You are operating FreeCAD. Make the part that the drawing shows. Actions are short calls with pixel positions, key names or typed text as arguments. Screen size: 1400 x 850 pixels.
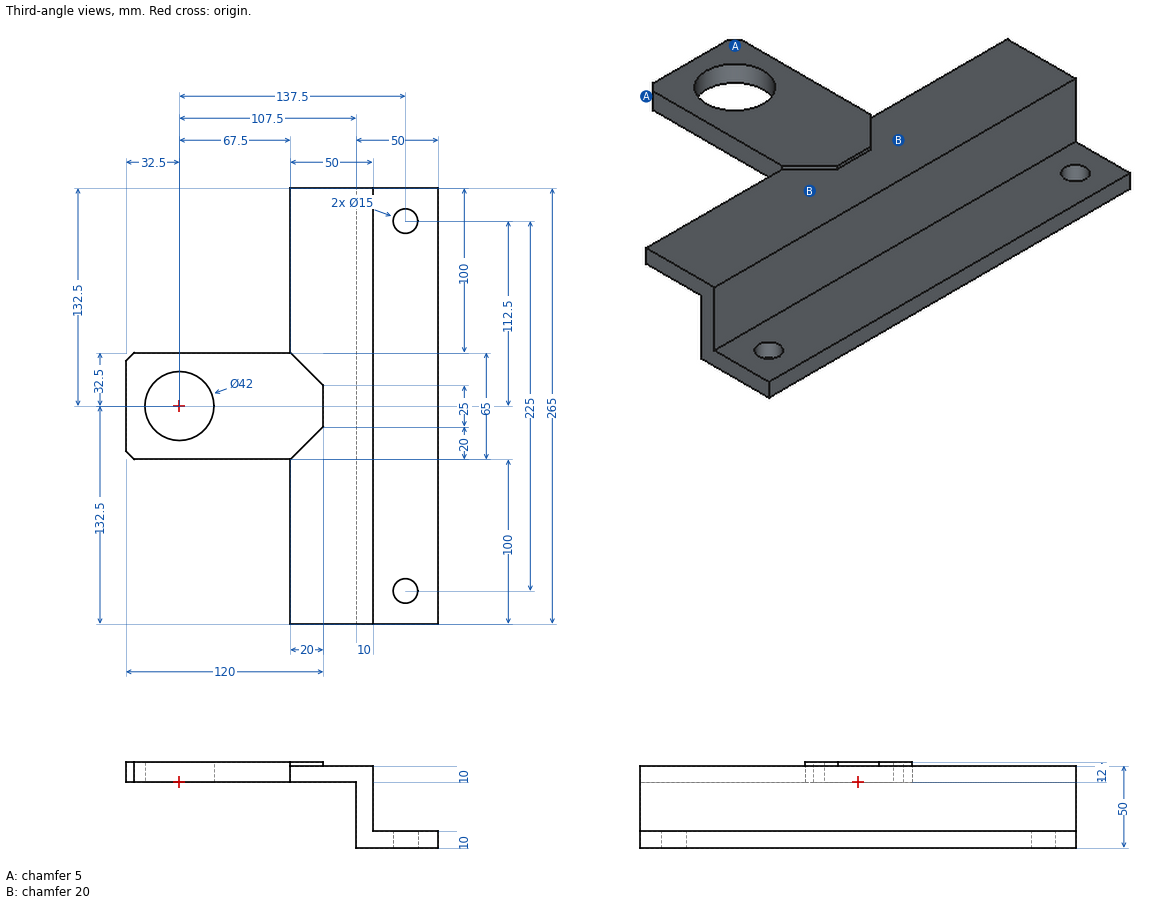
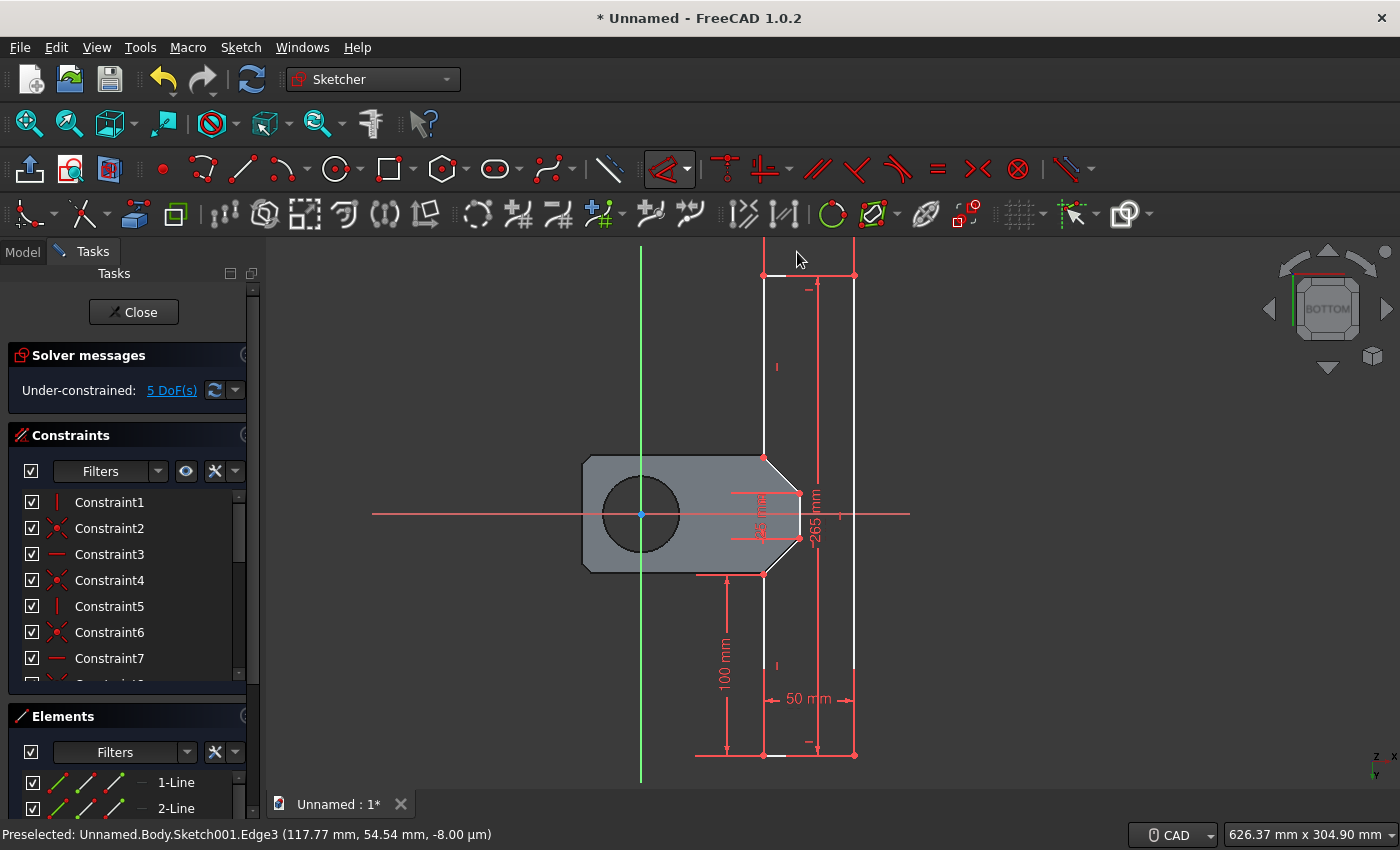
click(764, 330)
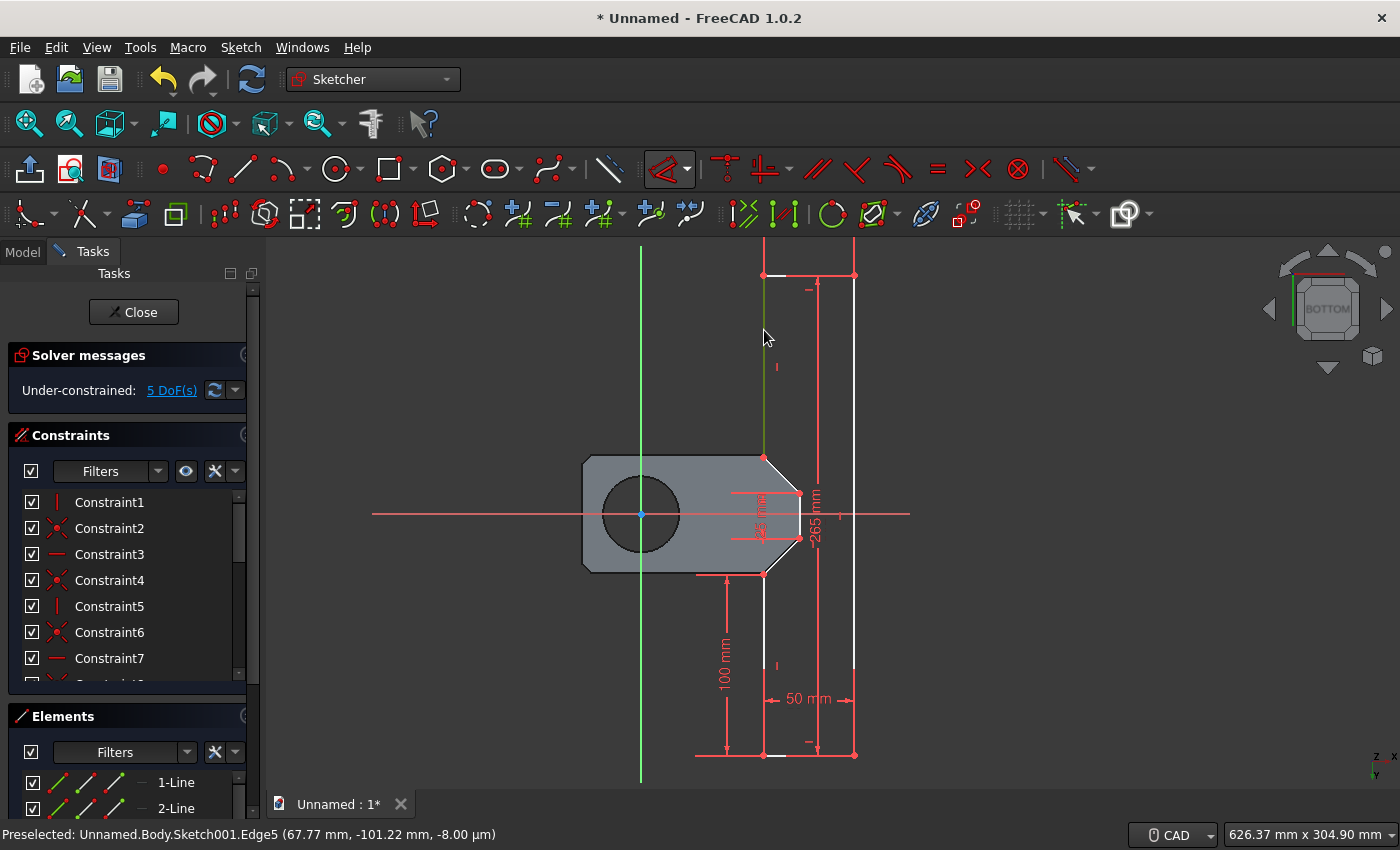
key(i)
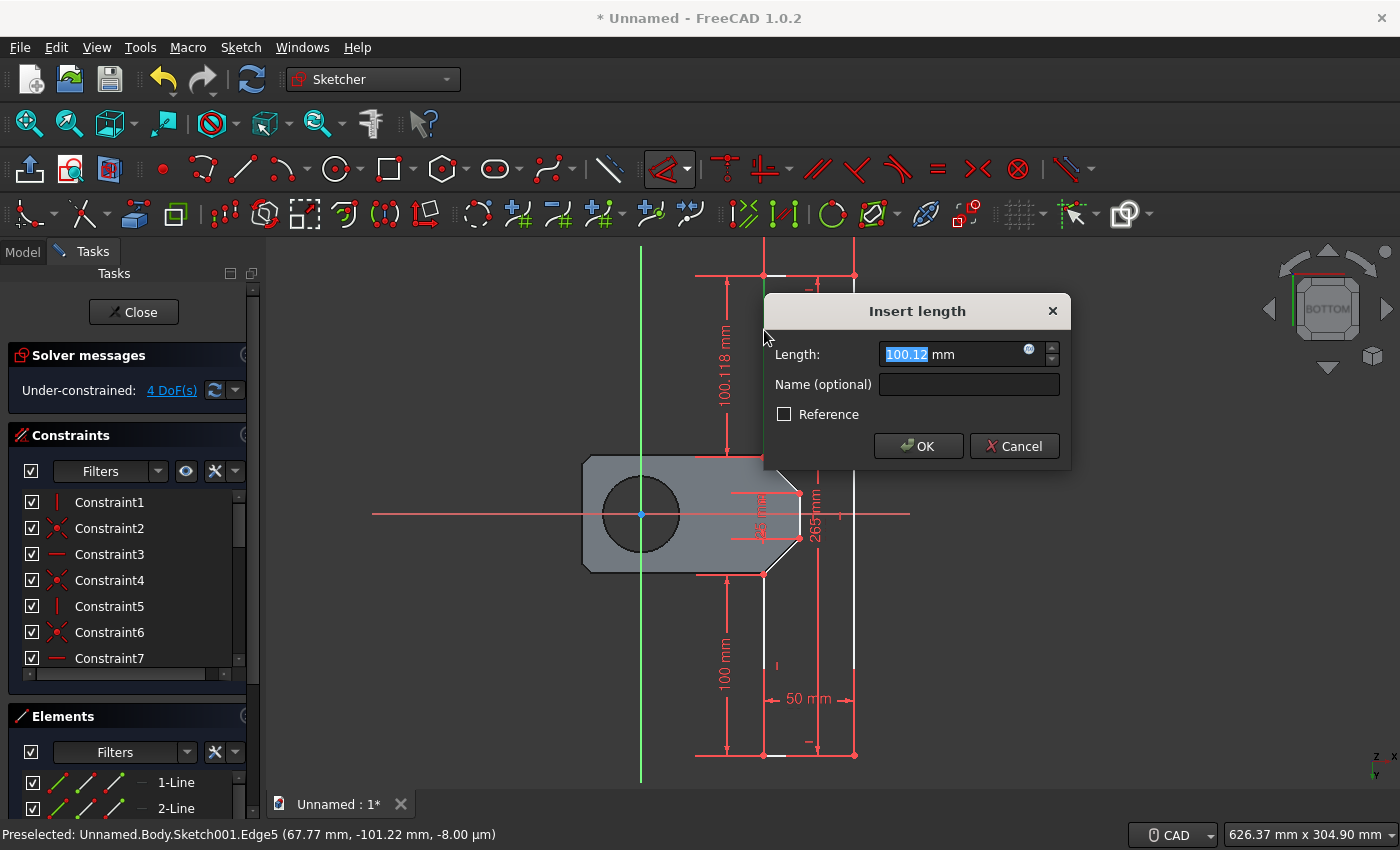
text(100)
key(Return)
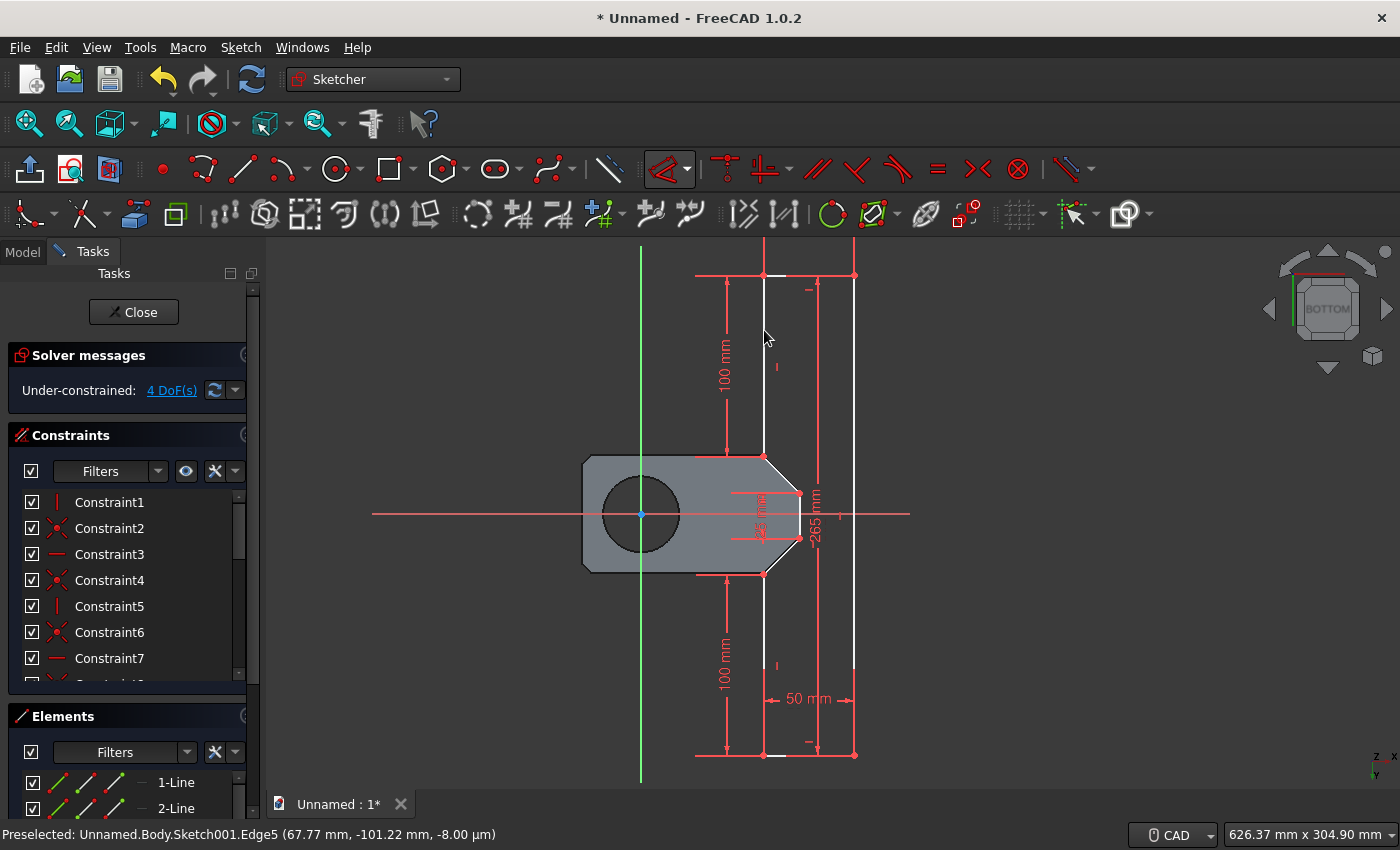
click(775, 468)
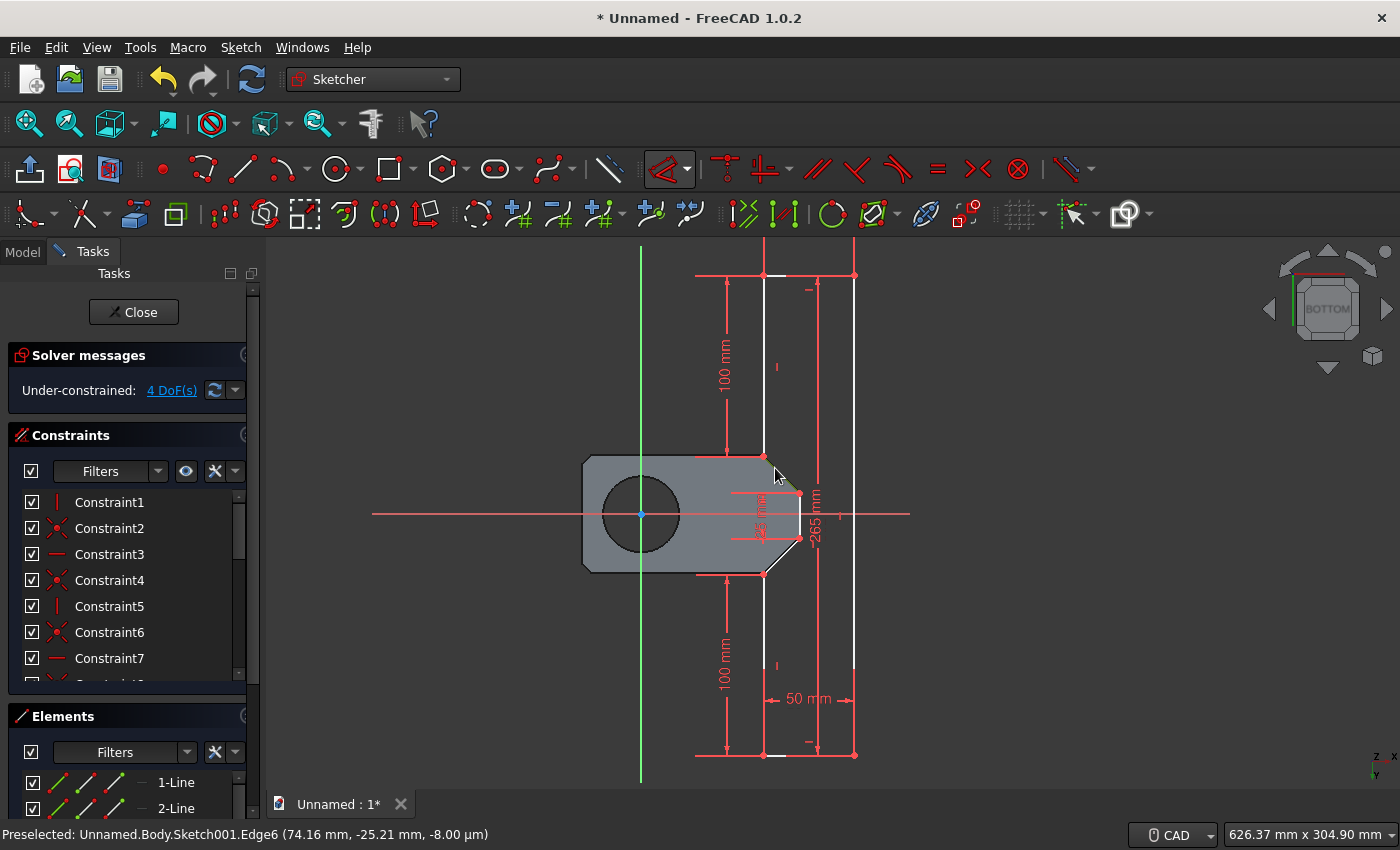
key(l)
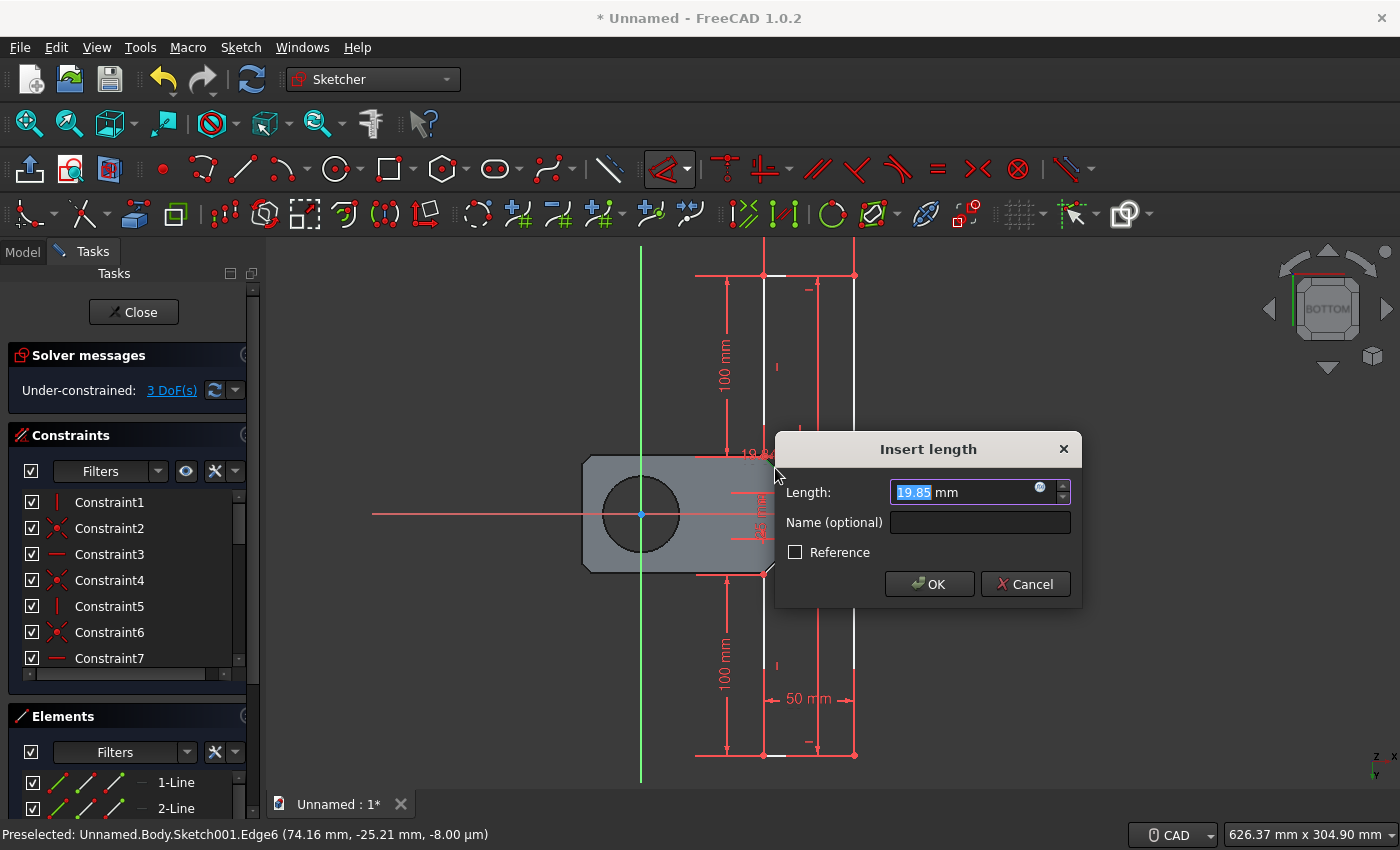
text(20)
key(Return)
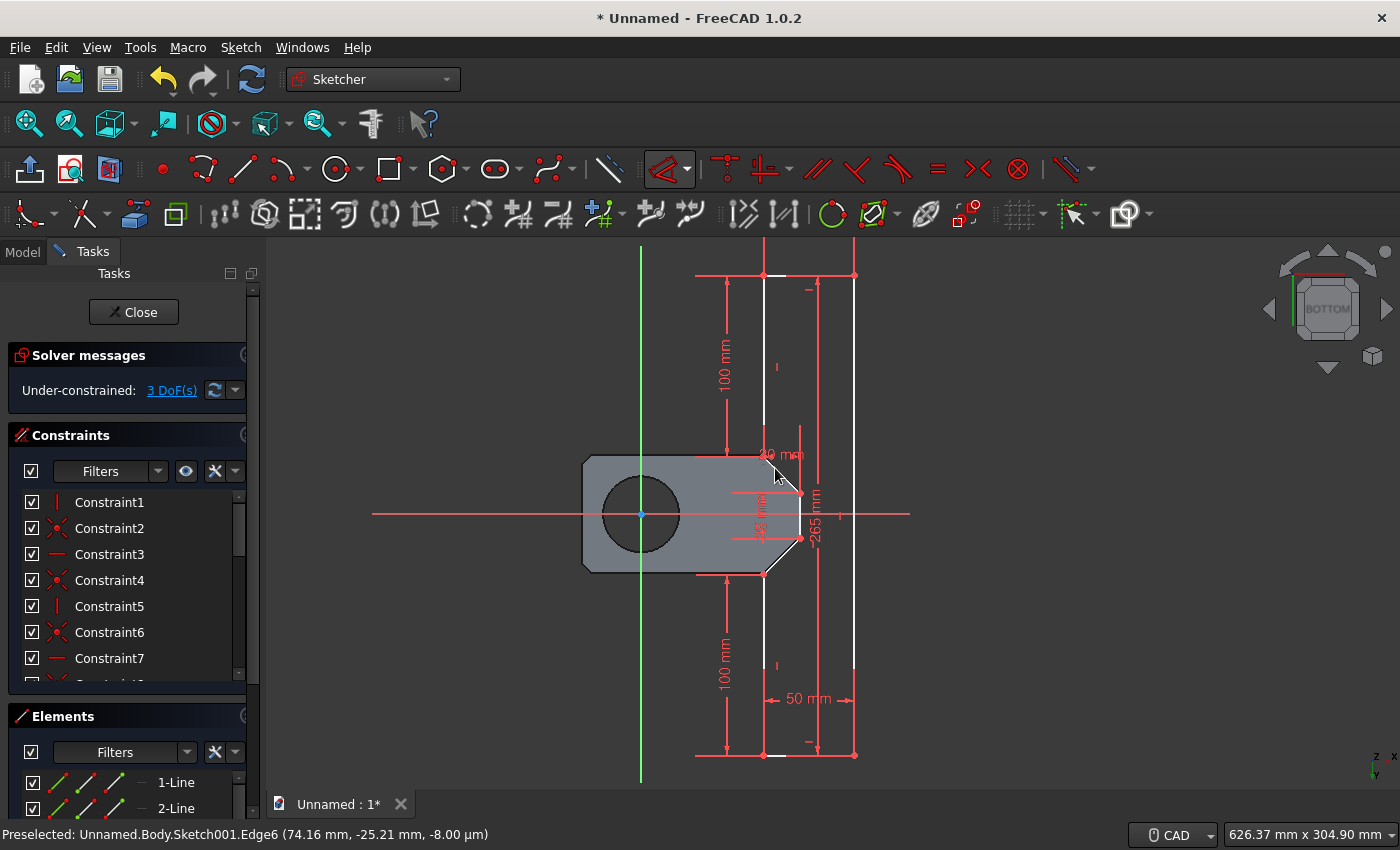
click(775, 468)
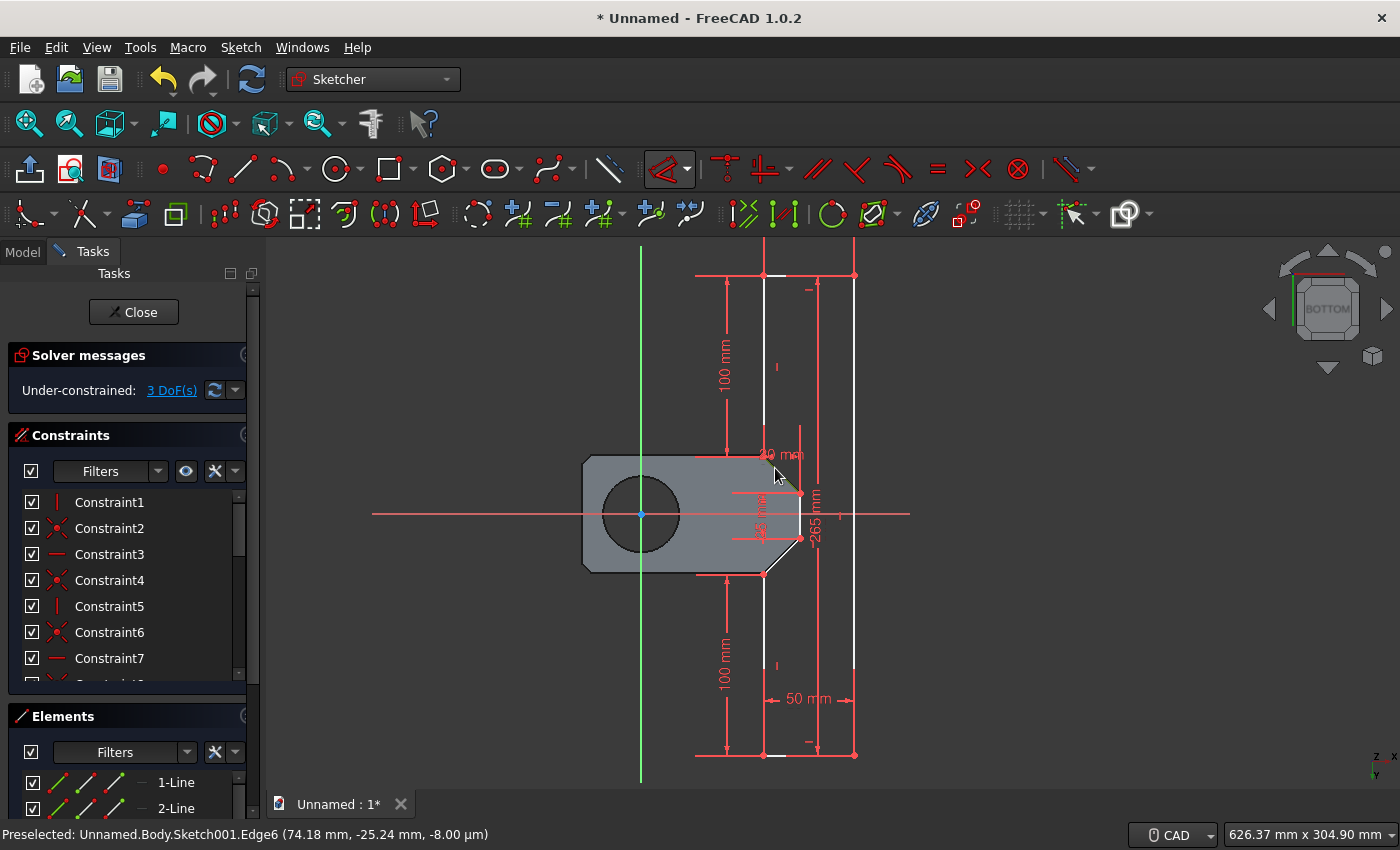
key(i)